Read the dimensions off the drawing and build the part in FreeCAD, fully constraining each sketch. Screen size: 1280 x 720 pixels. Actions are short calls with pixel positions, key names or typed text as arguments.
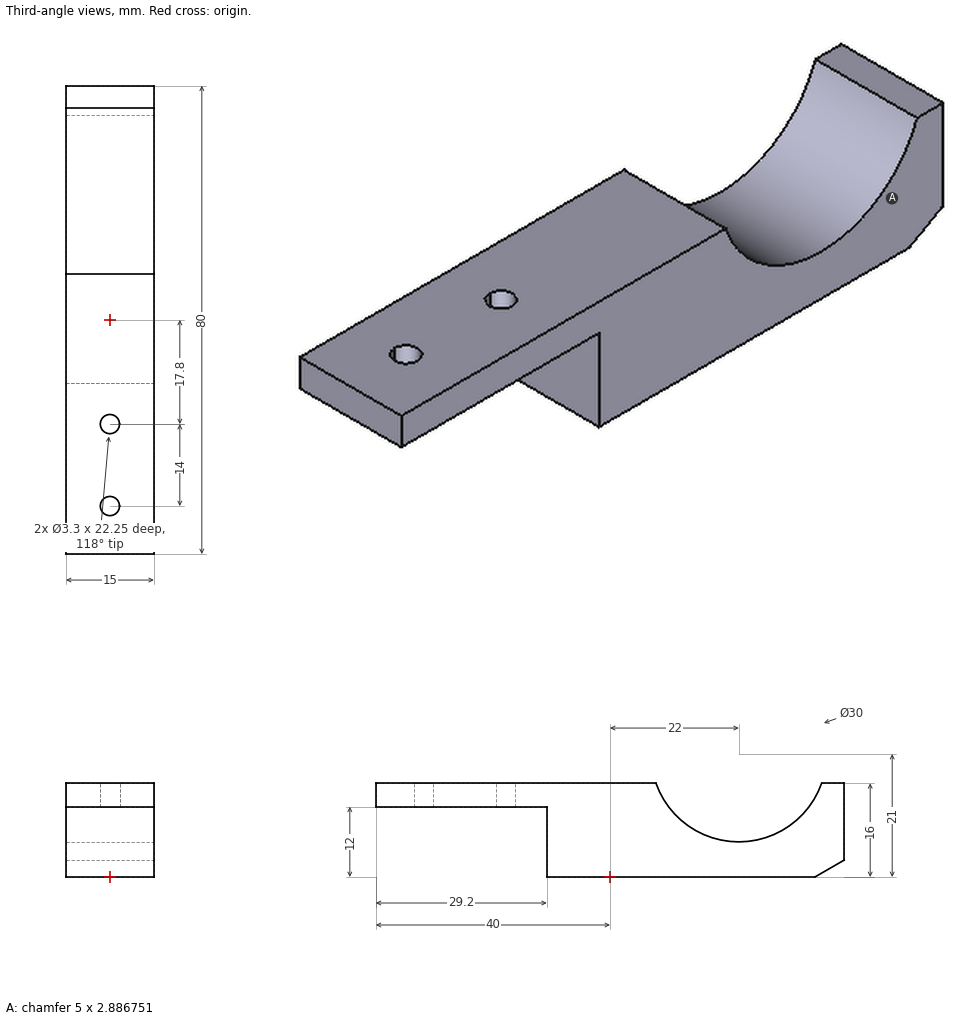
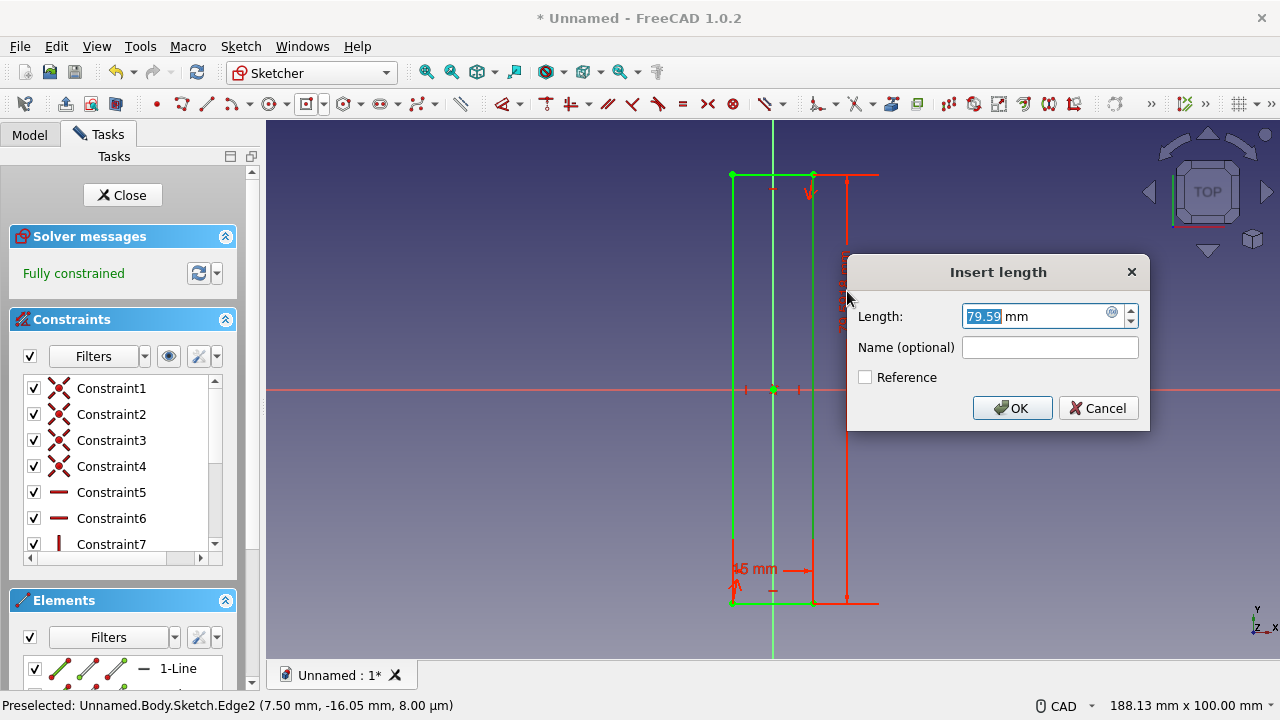
text(80)
key(Return)
key(Escape)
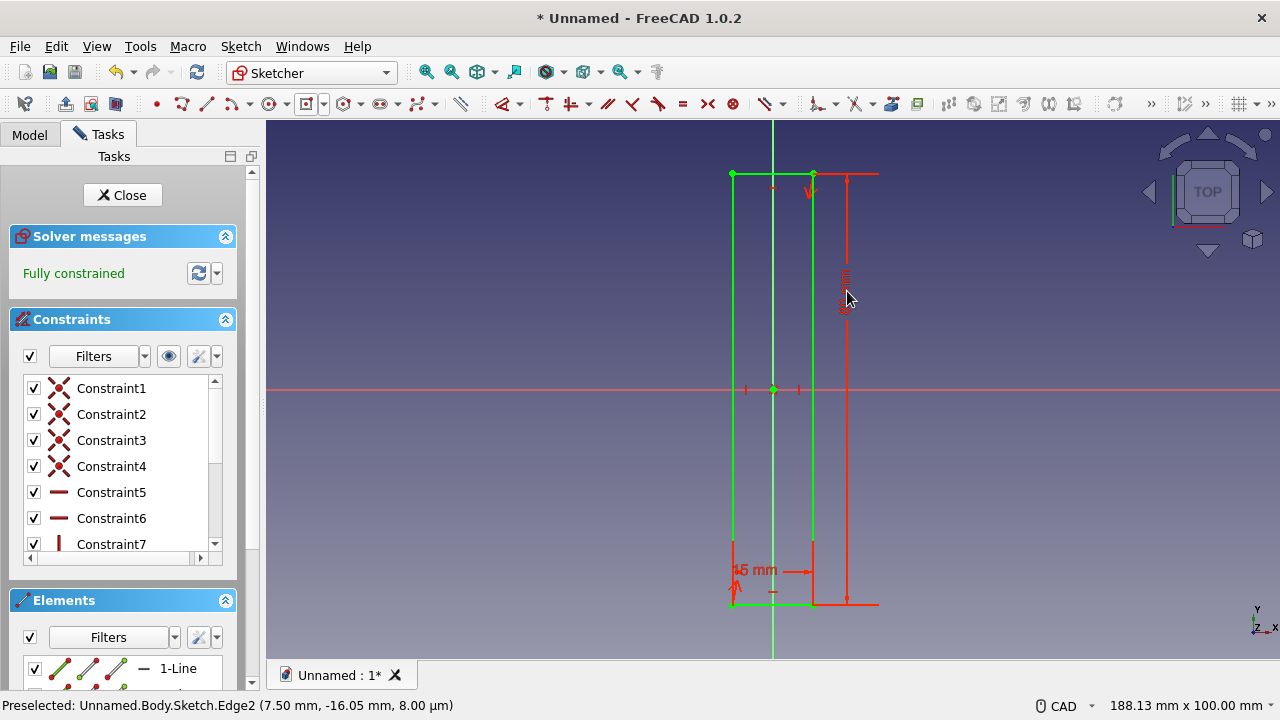
click(123, 195)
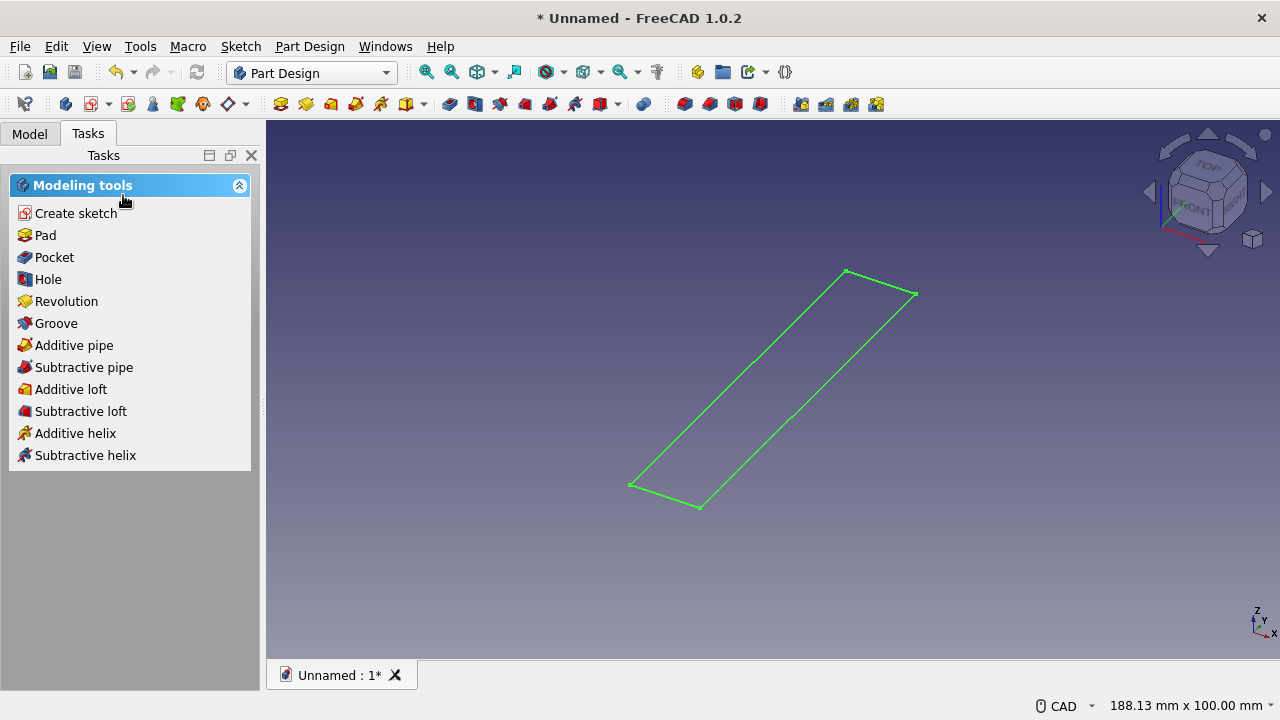
click(281, 104)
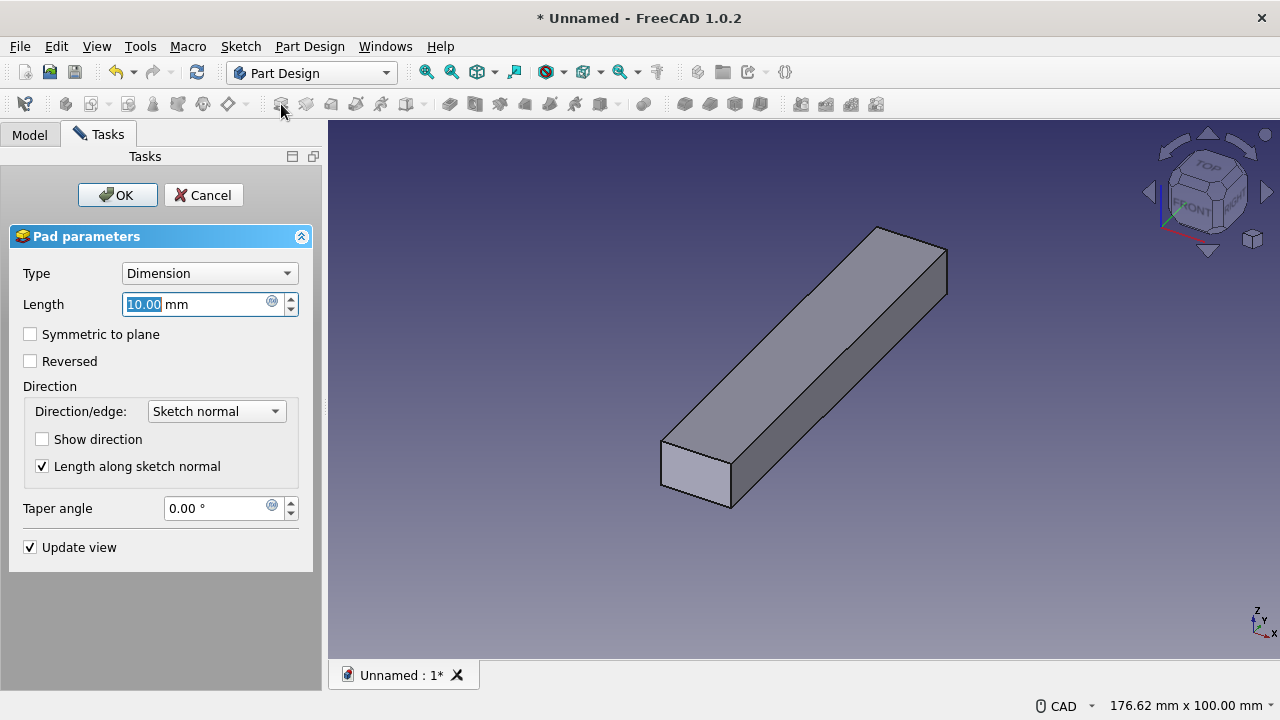
text(16)
key(Tab)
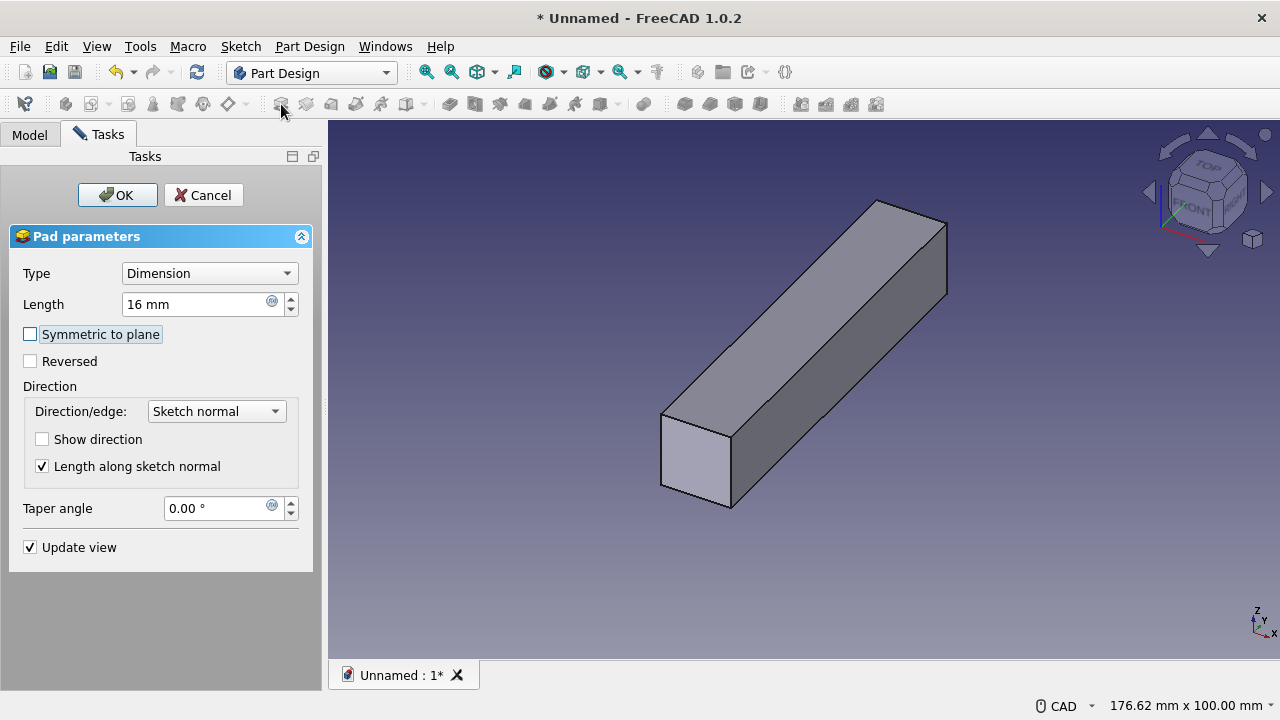
click(118, 195)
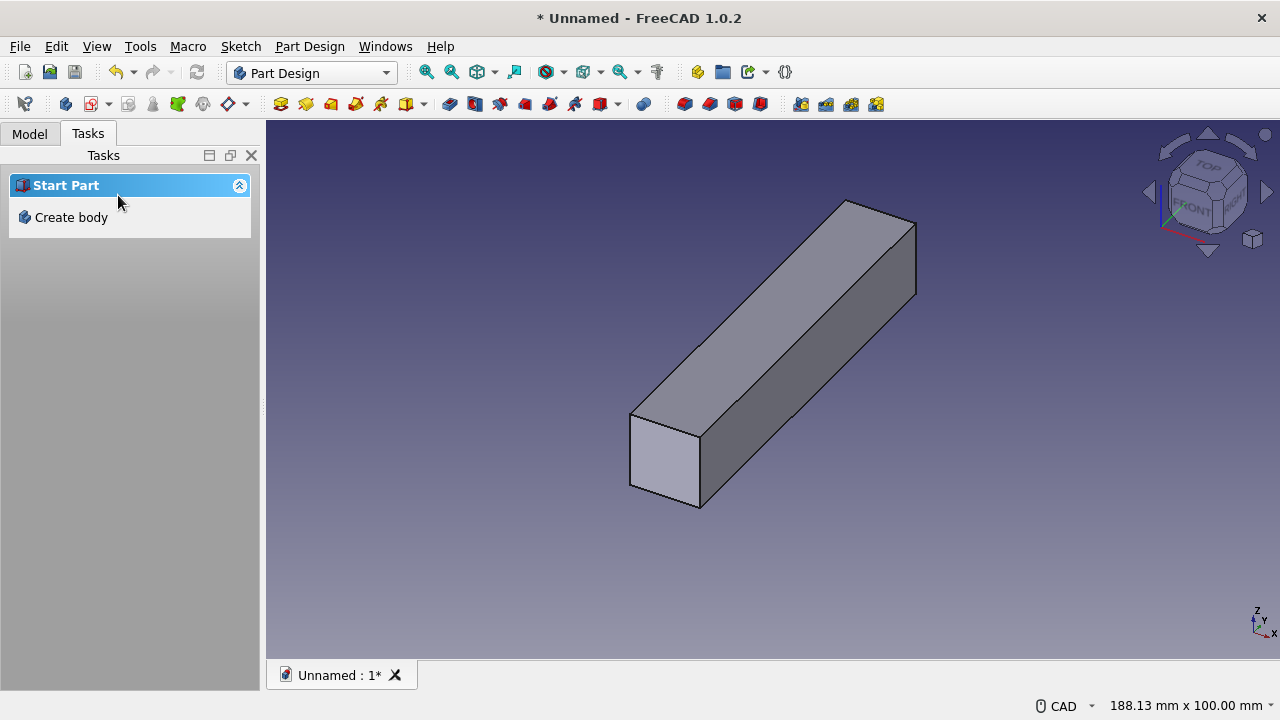
click(870, 304)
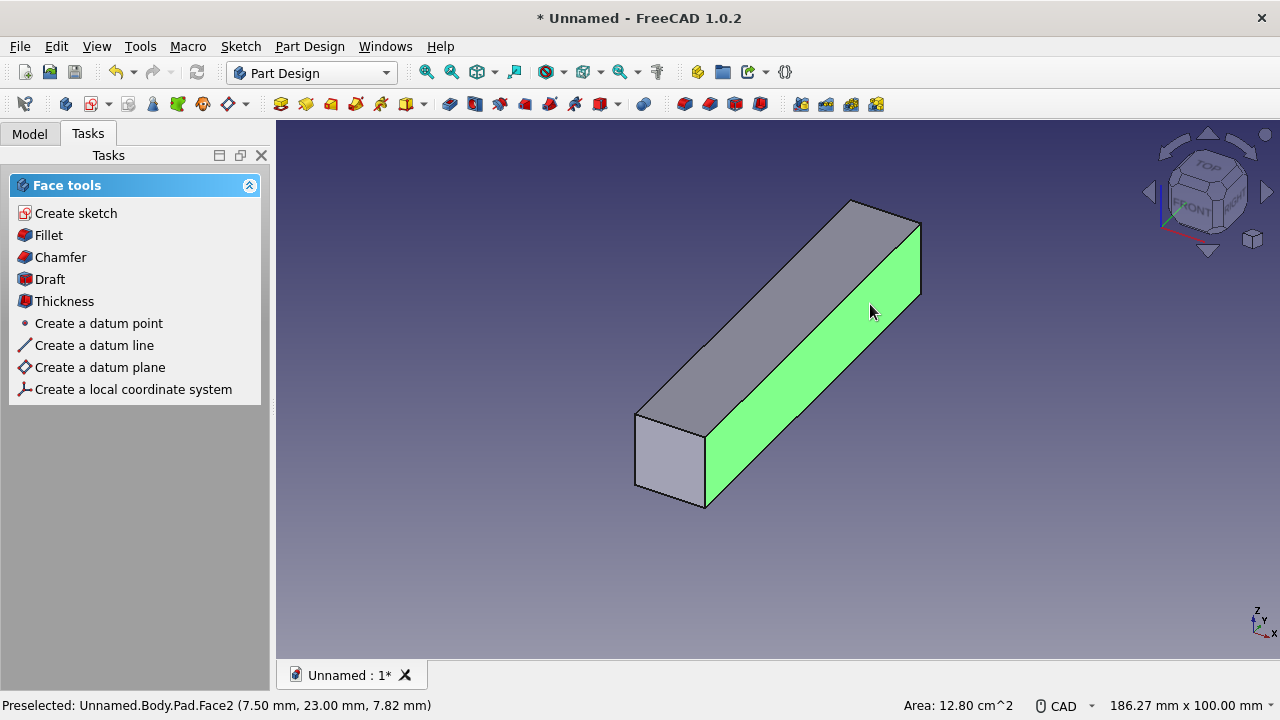
click(90, 104)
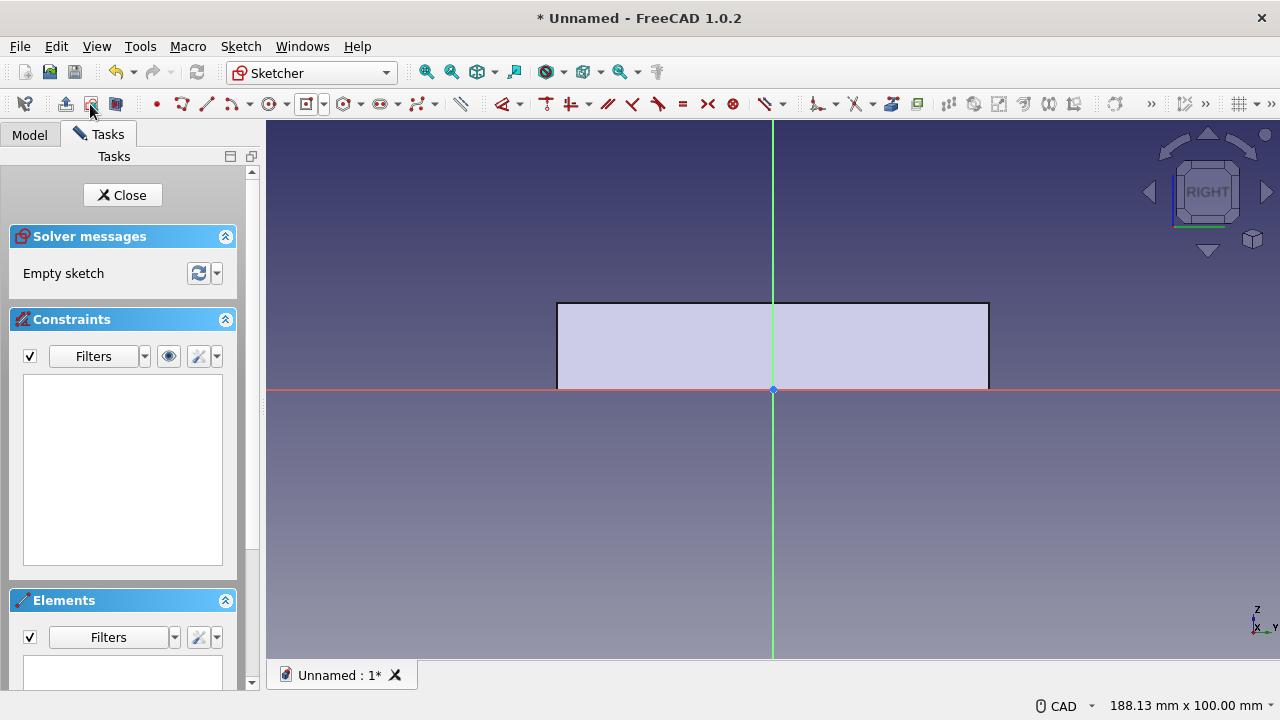
scroll(642, 338, up, 5)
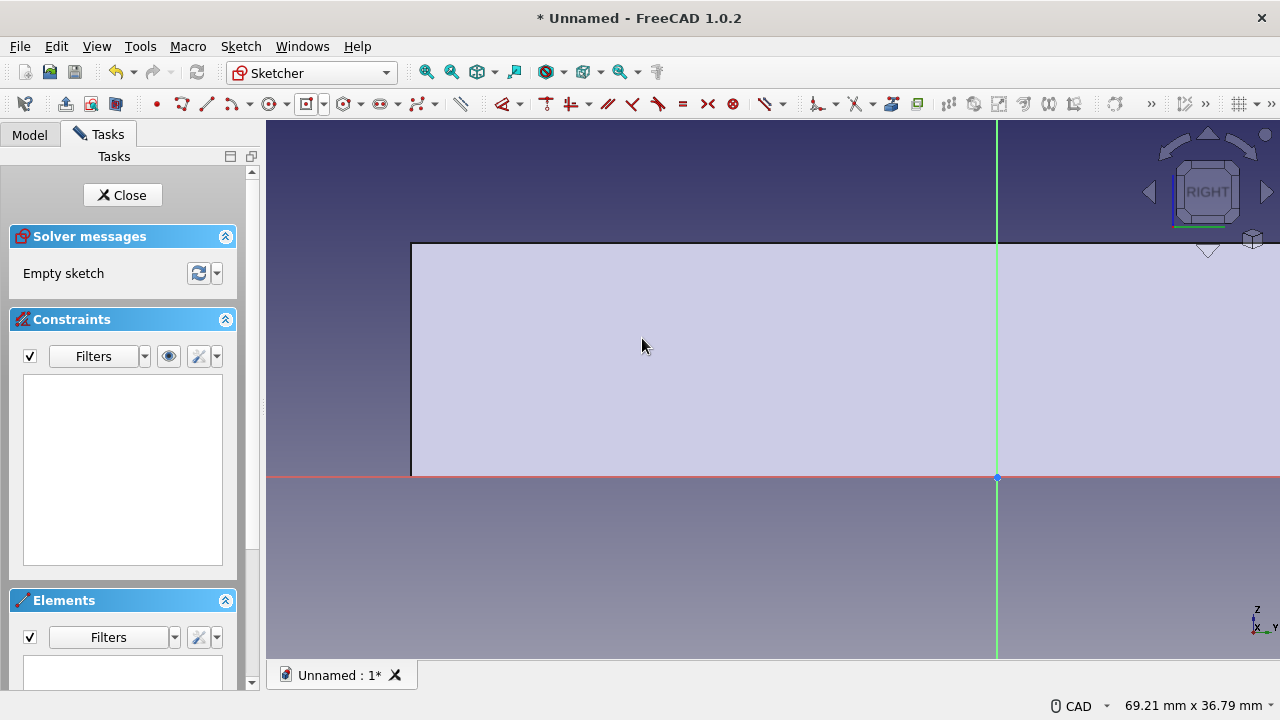
key(g)
key(r)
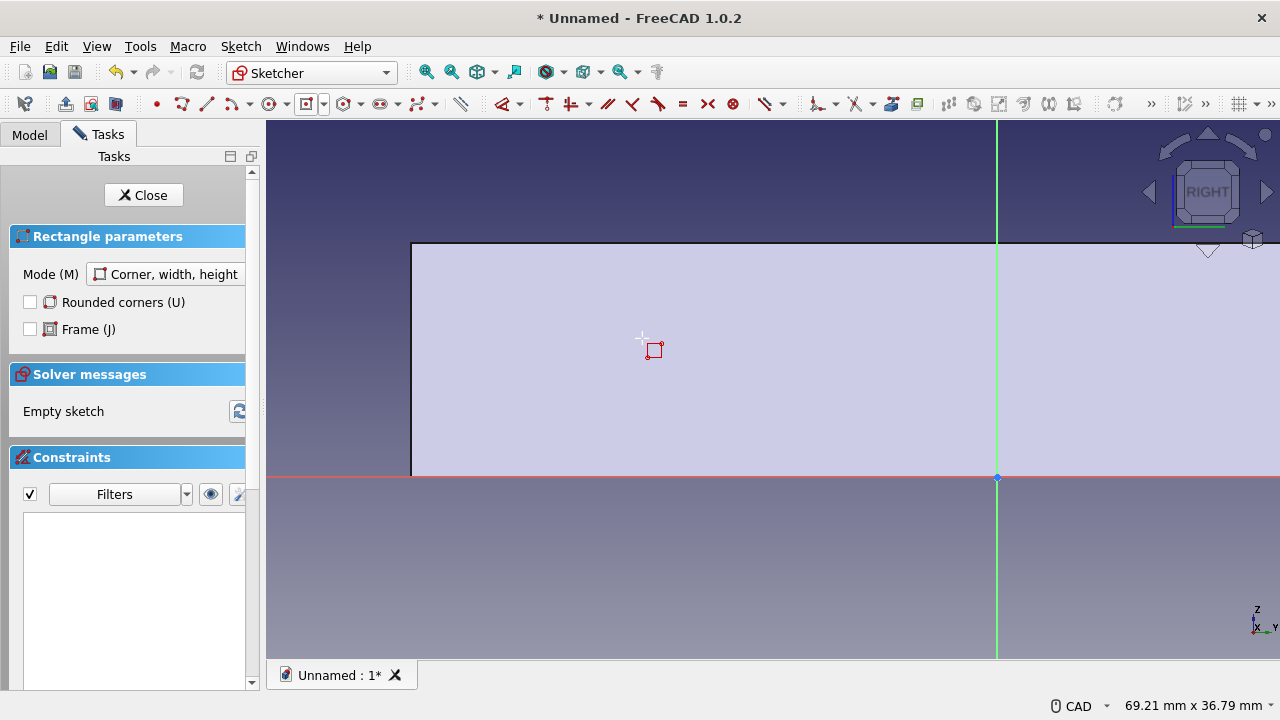
click(411, 301)
click(839, 477)
key(Escape)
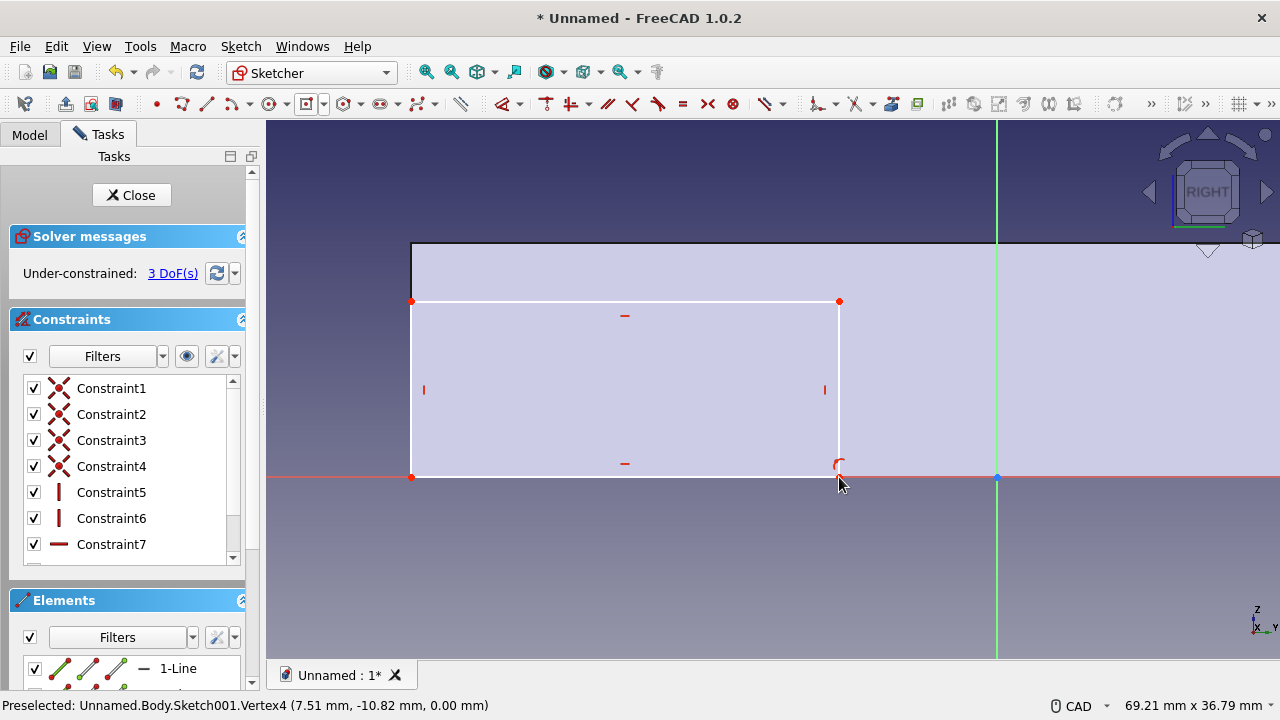
click(502, 104)